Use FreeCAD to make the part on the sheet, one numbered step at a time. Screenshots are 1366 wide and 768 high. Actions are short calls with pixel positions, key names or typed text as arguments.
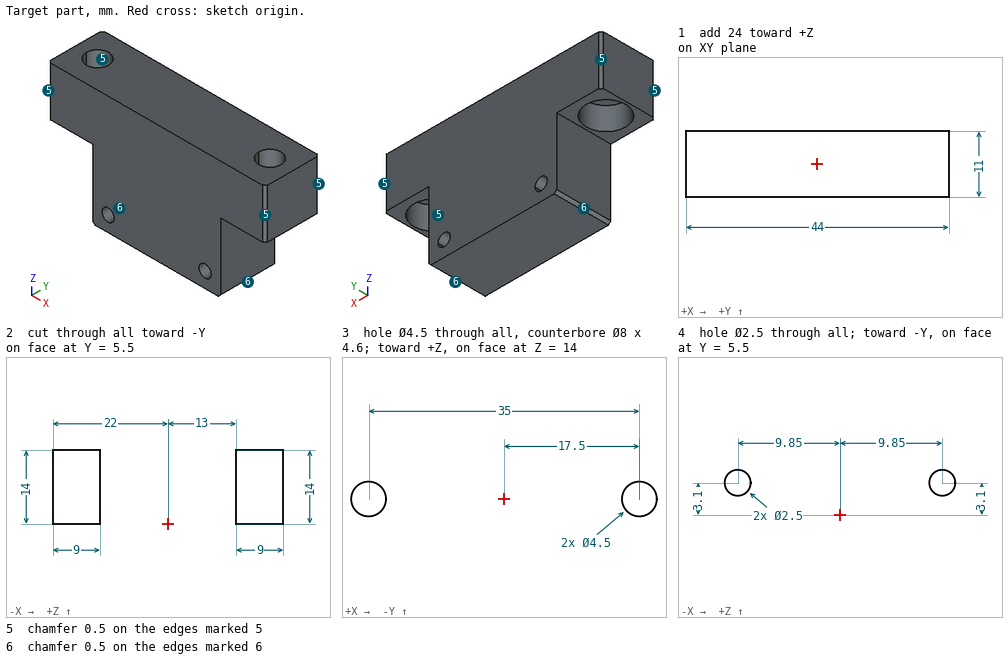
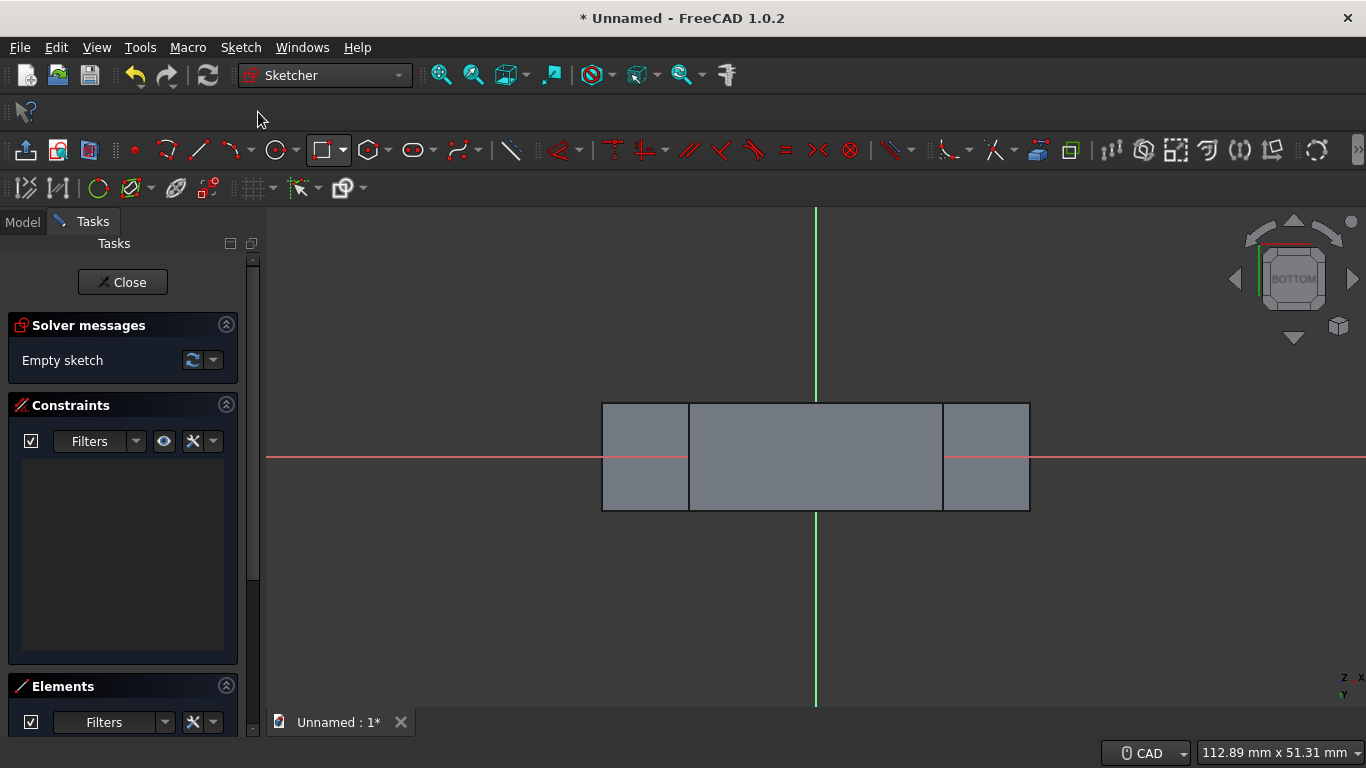
scroll(899, 457, up, 3)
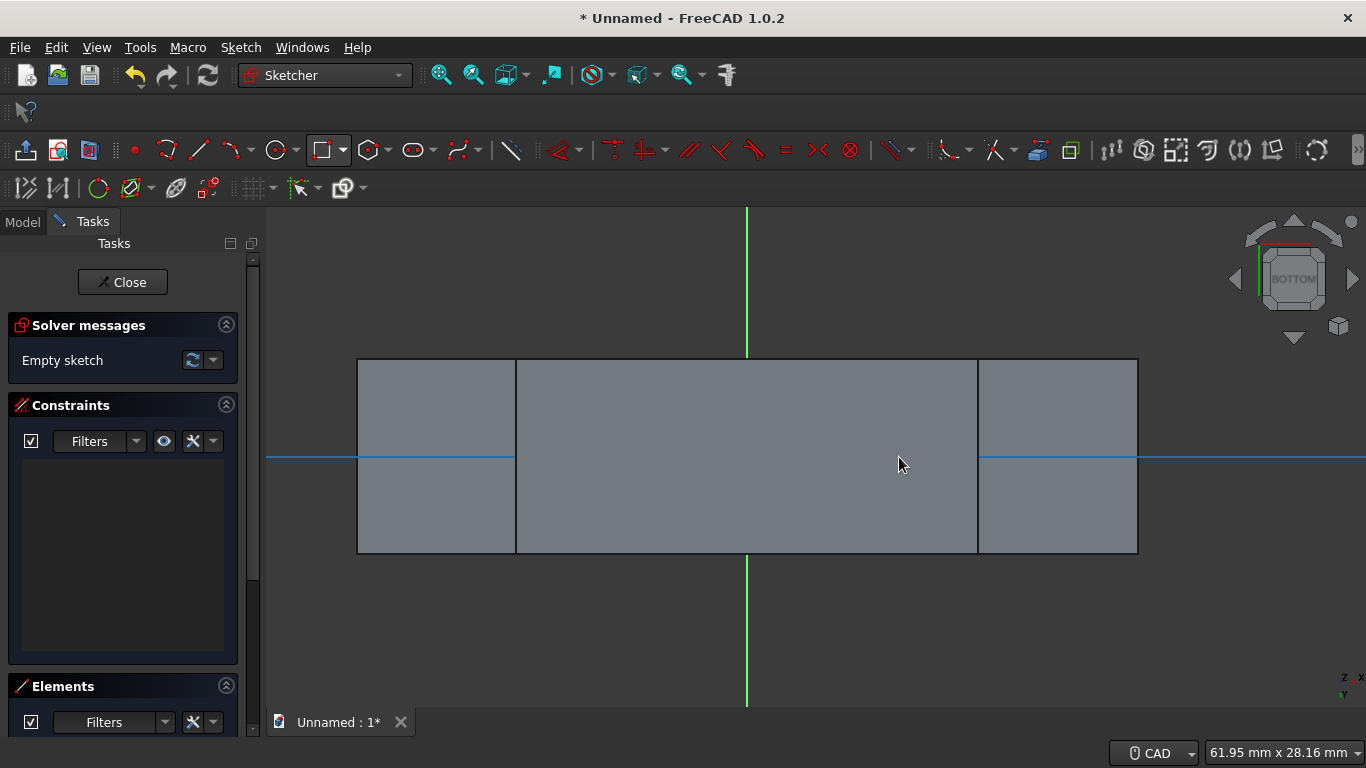
click(276, 150)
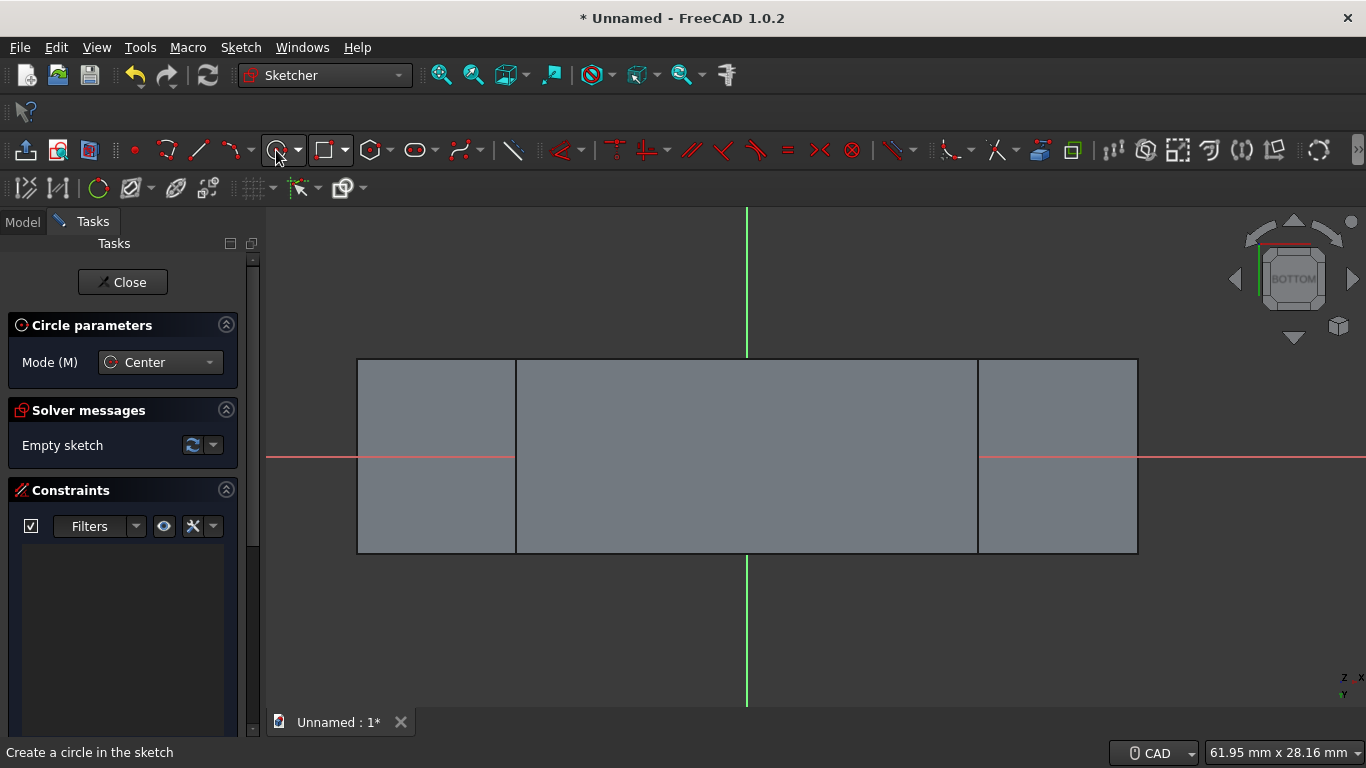
click(1058, 457)
move(1086, 428)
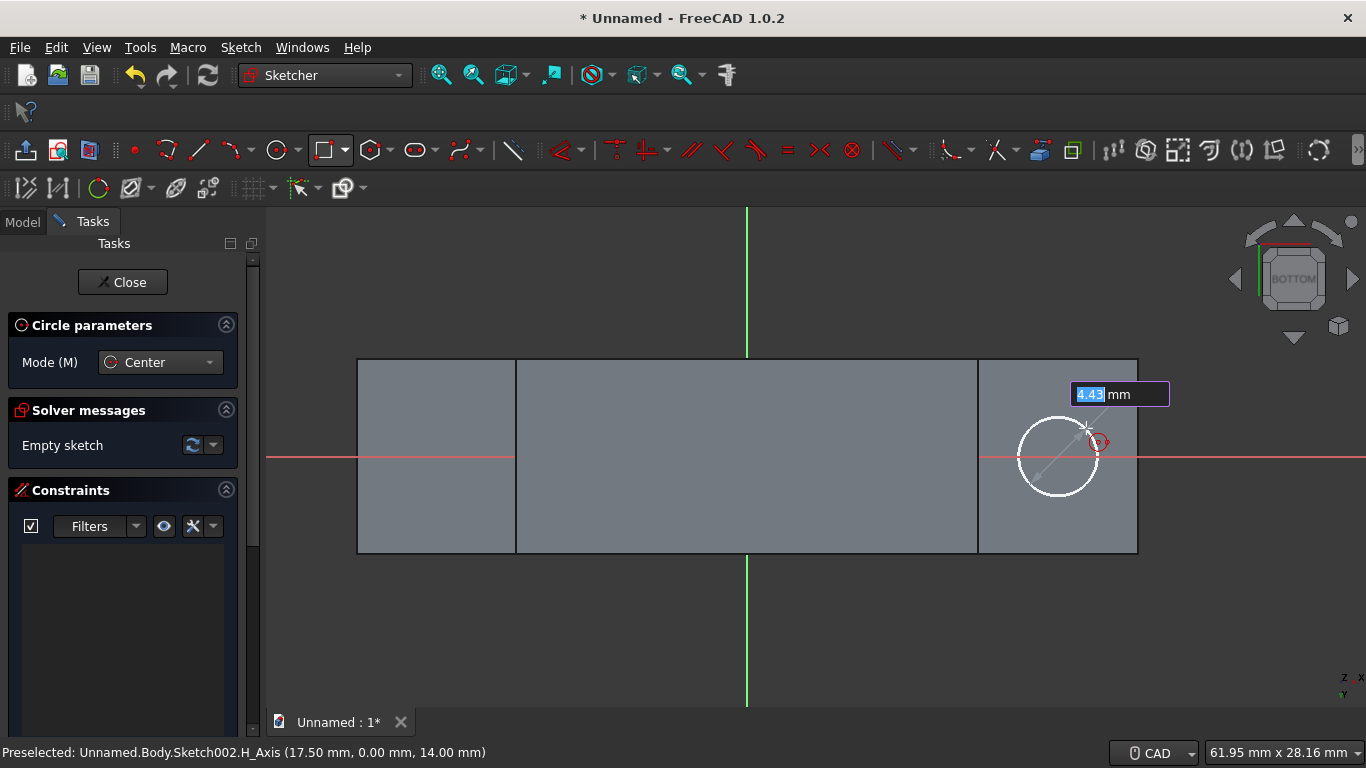
text(4.5)
key(Return)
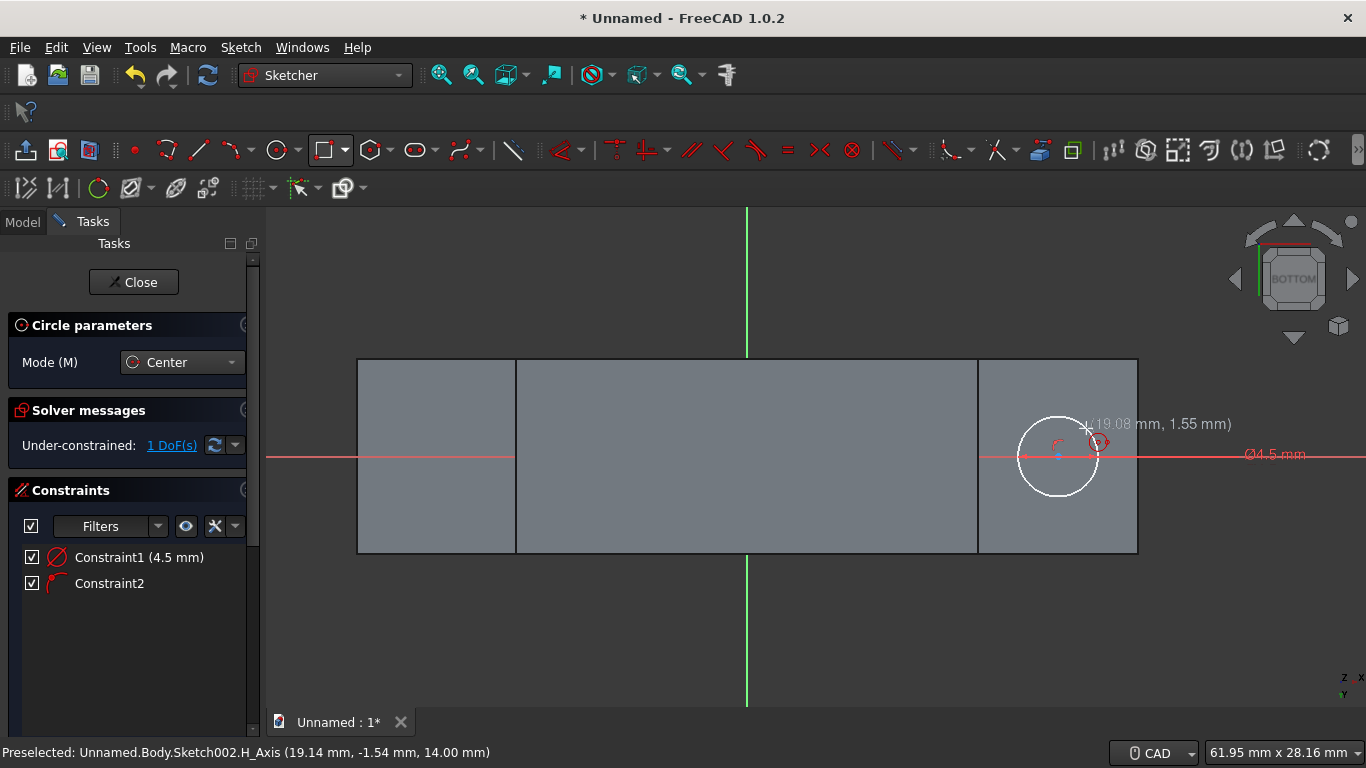
click(437, 457)
move(465, 428)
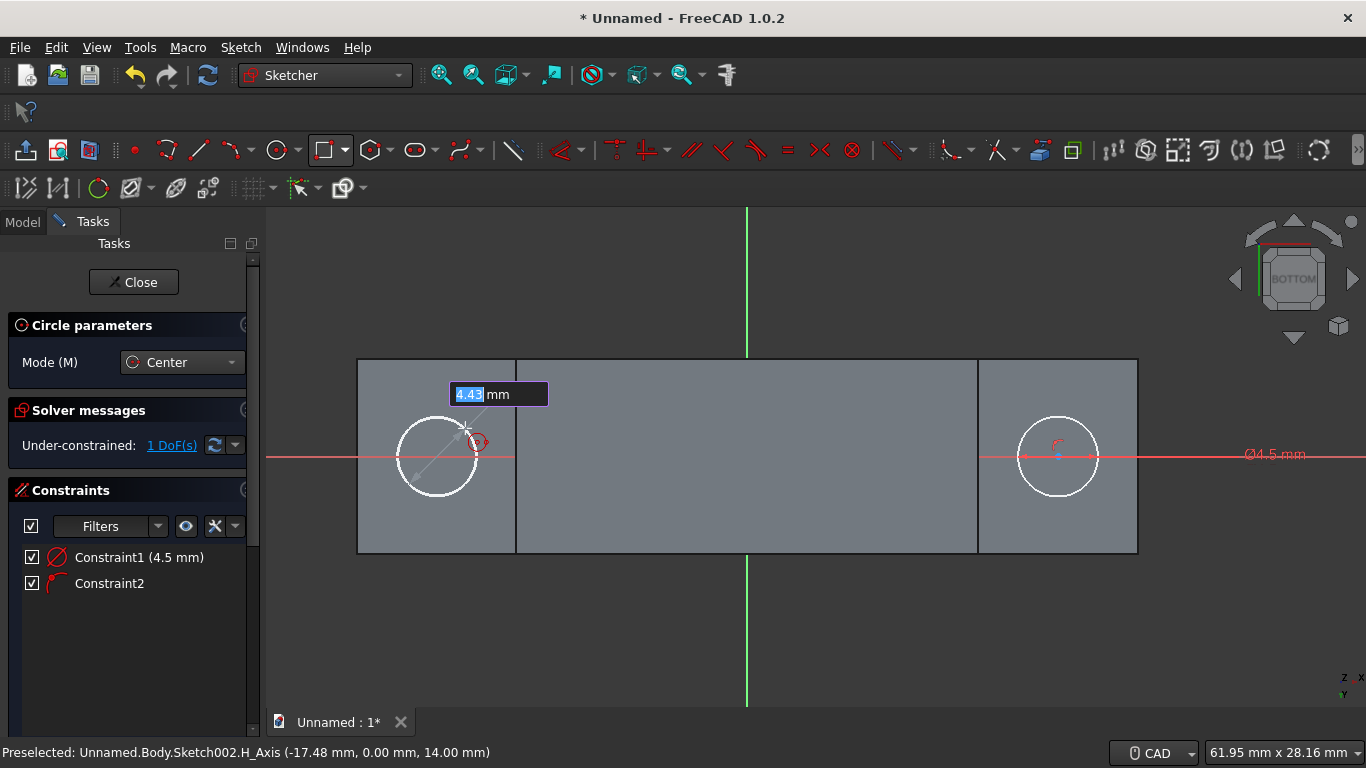
text(4.5)
key(Return)
key(Escape)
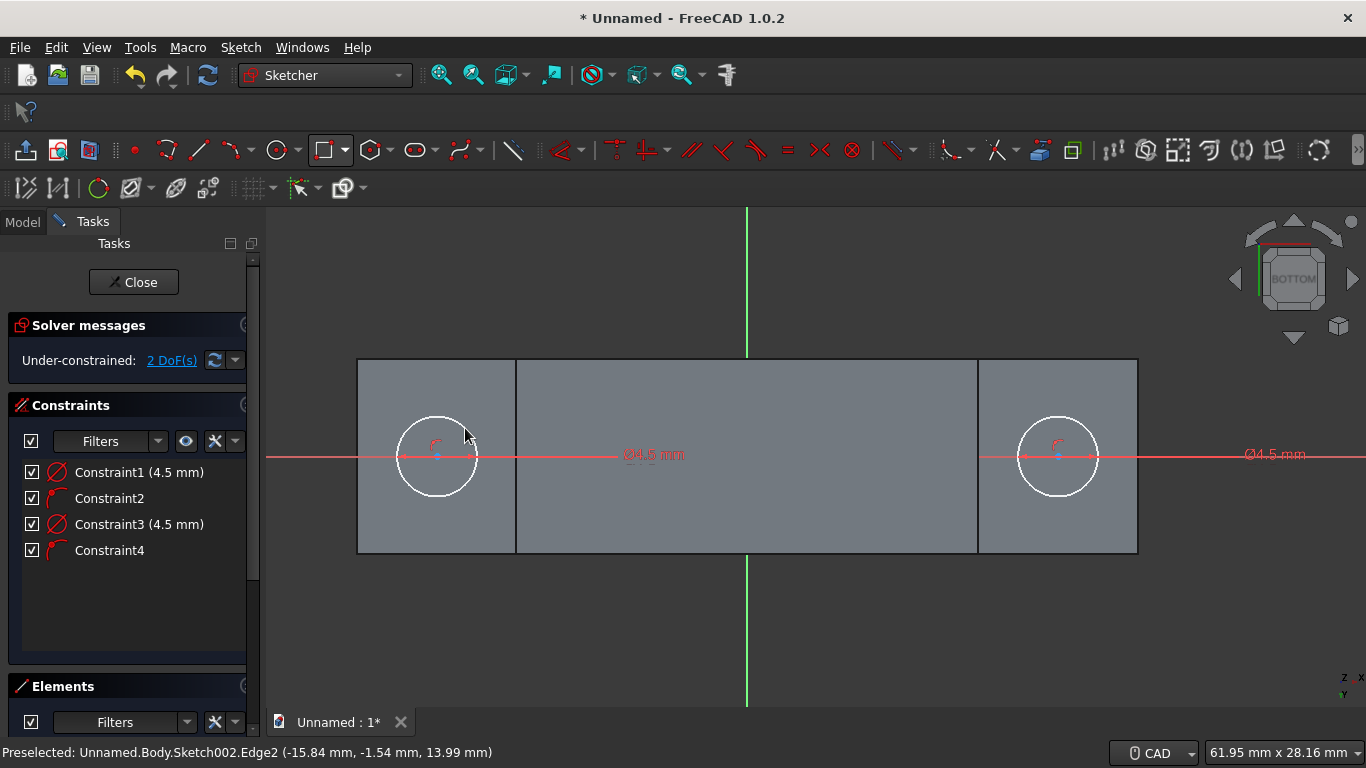
click(560, 150)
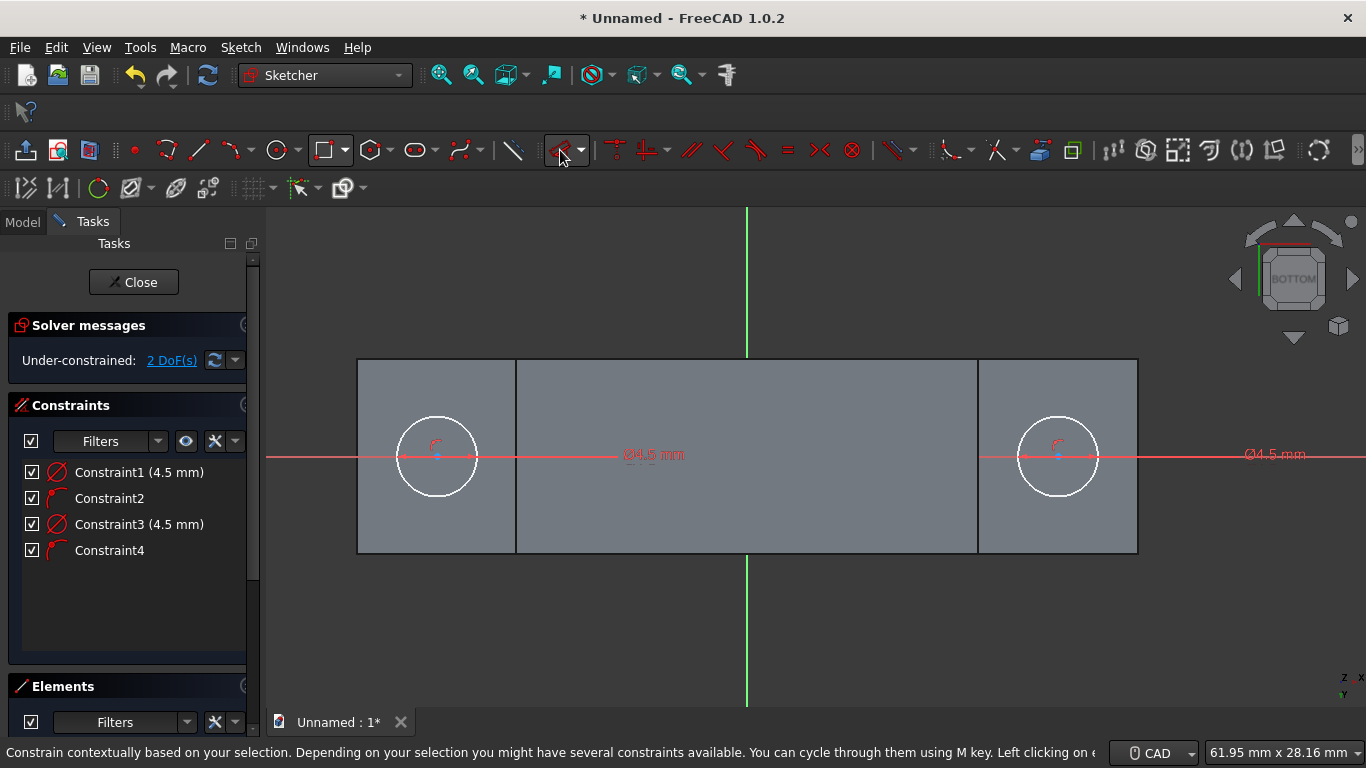
click(1058, 457)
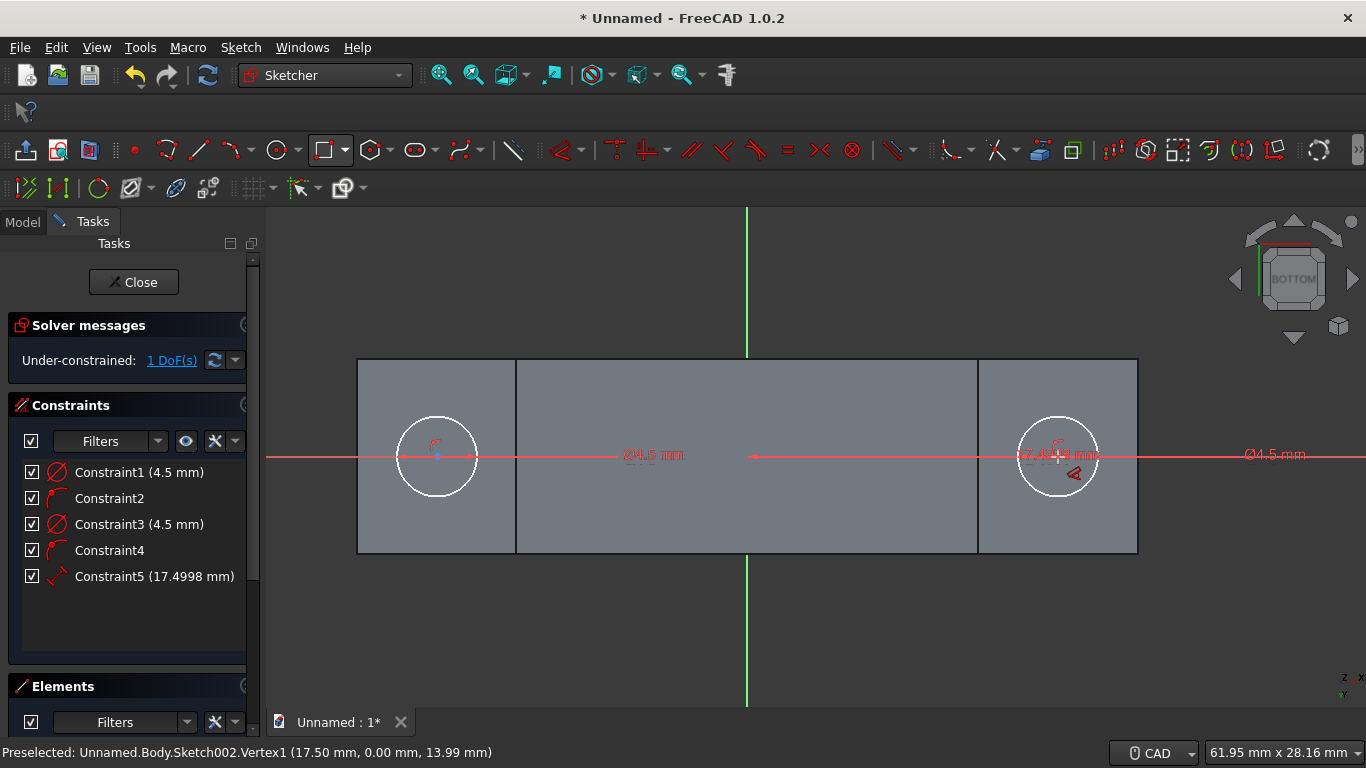
click(437, 457)
click(605, 491)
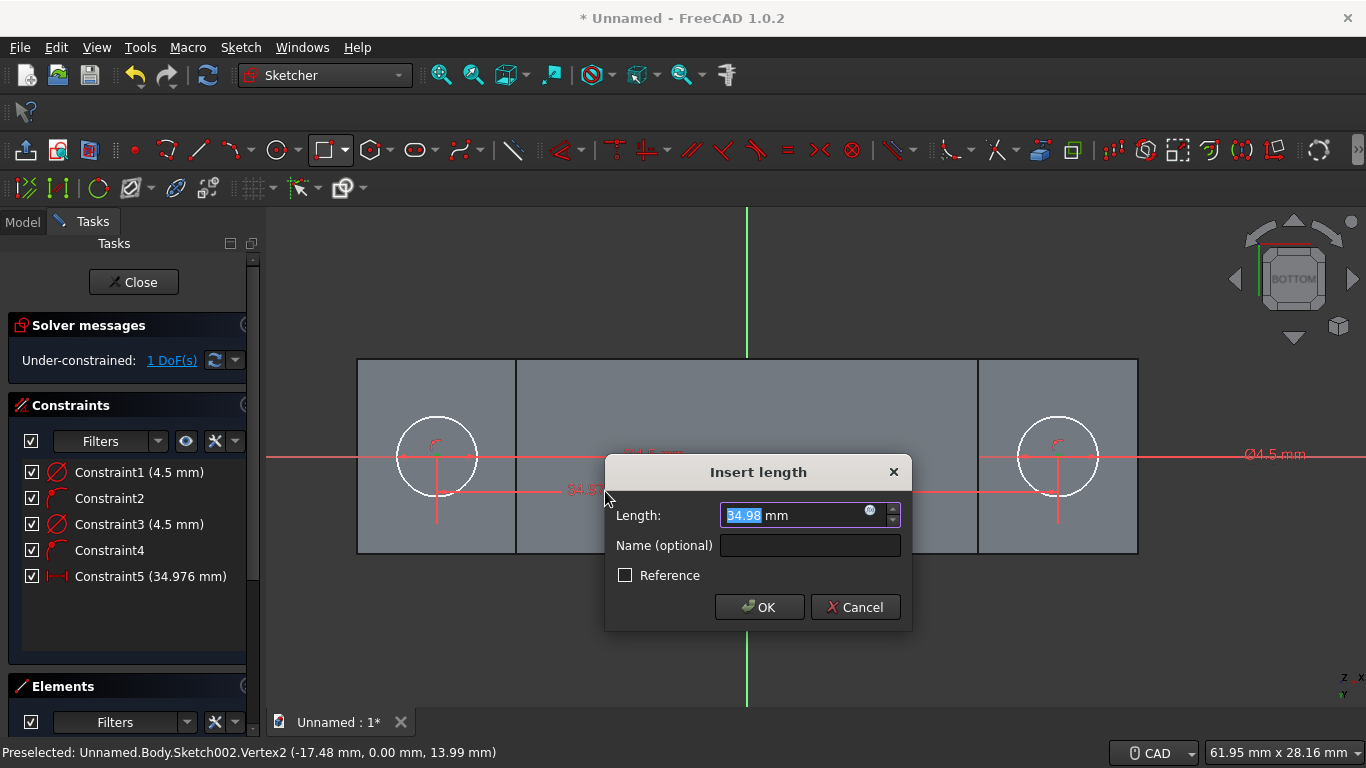
text(35)
key(Return)